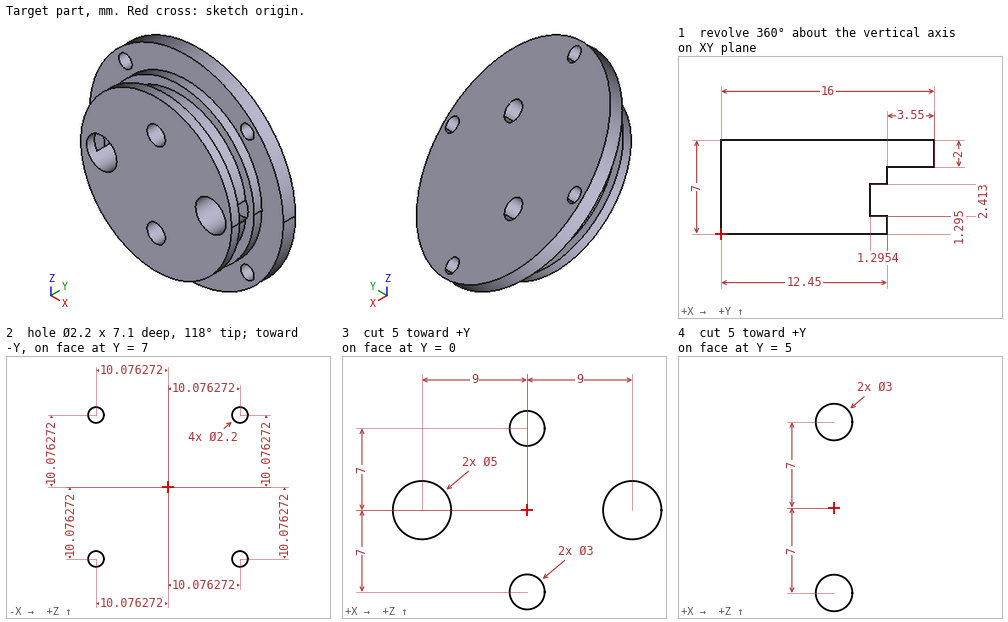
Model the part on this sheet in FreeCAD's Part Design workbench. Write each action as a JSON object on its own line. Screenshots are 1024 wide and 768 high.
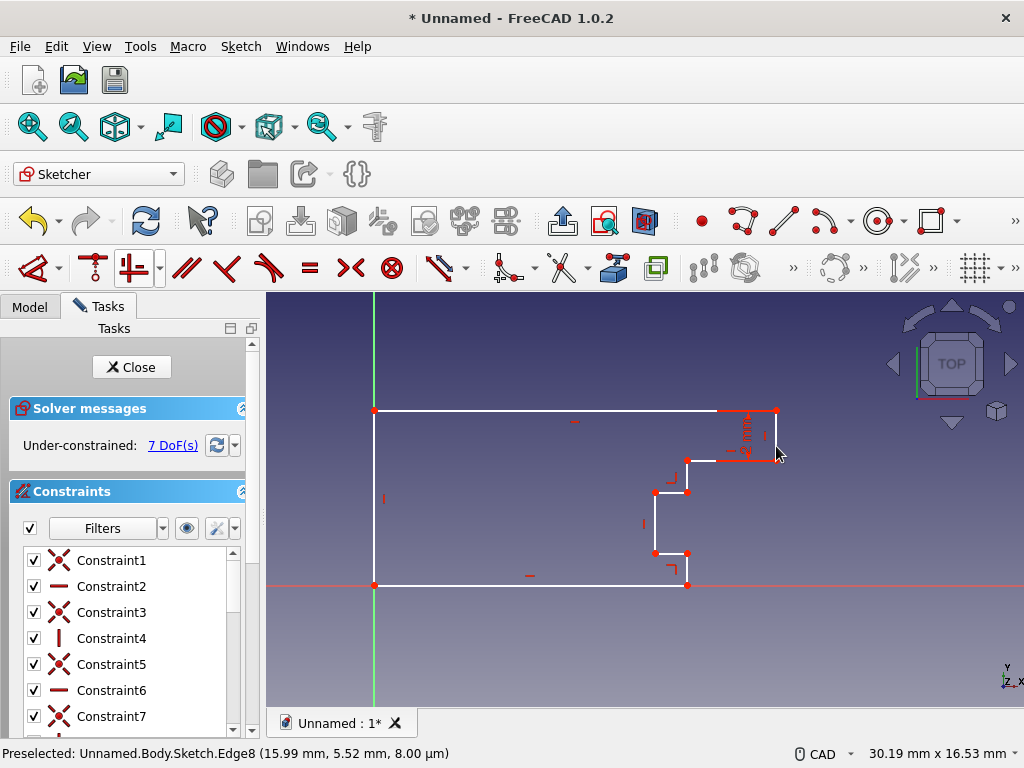
{"action": "left_click", "coordinate": [374, 463]}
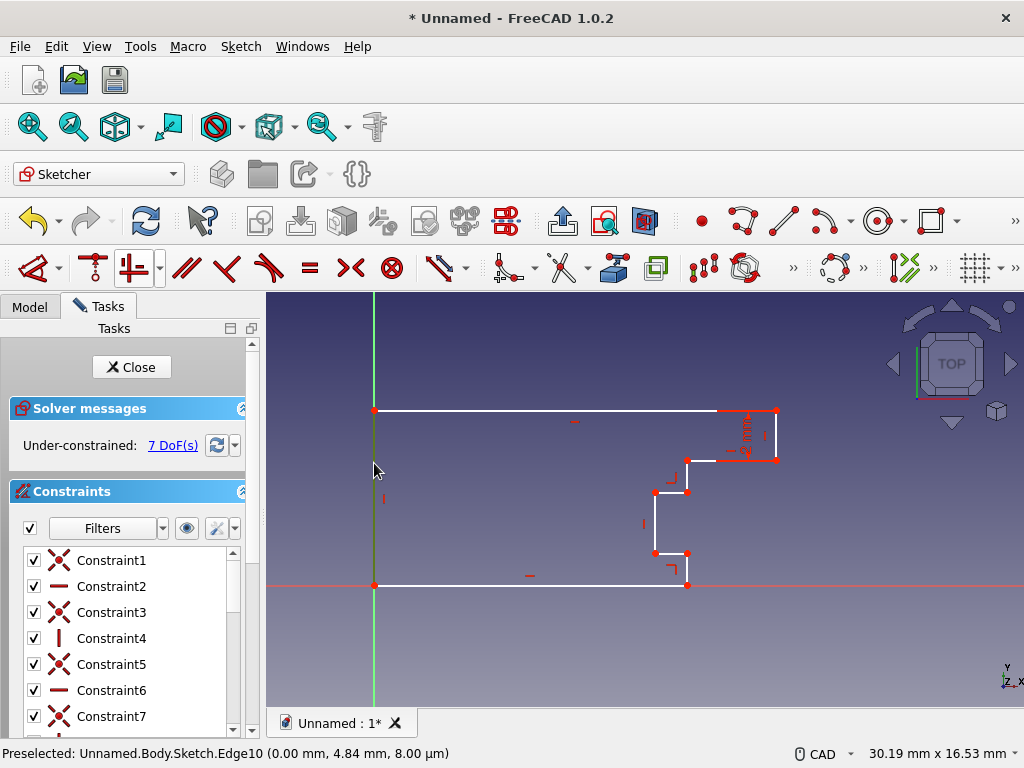
{"action": "left_click", "coordinate": [58, 268]}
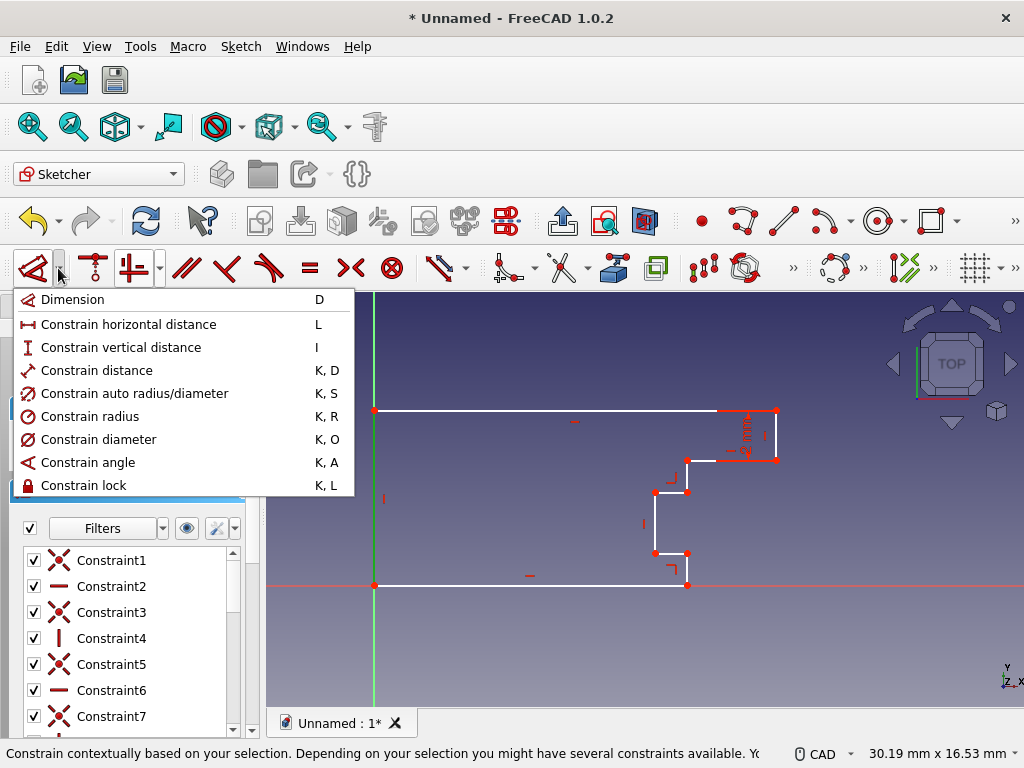
{"action": "left_click", "coordinate": [184, 348]}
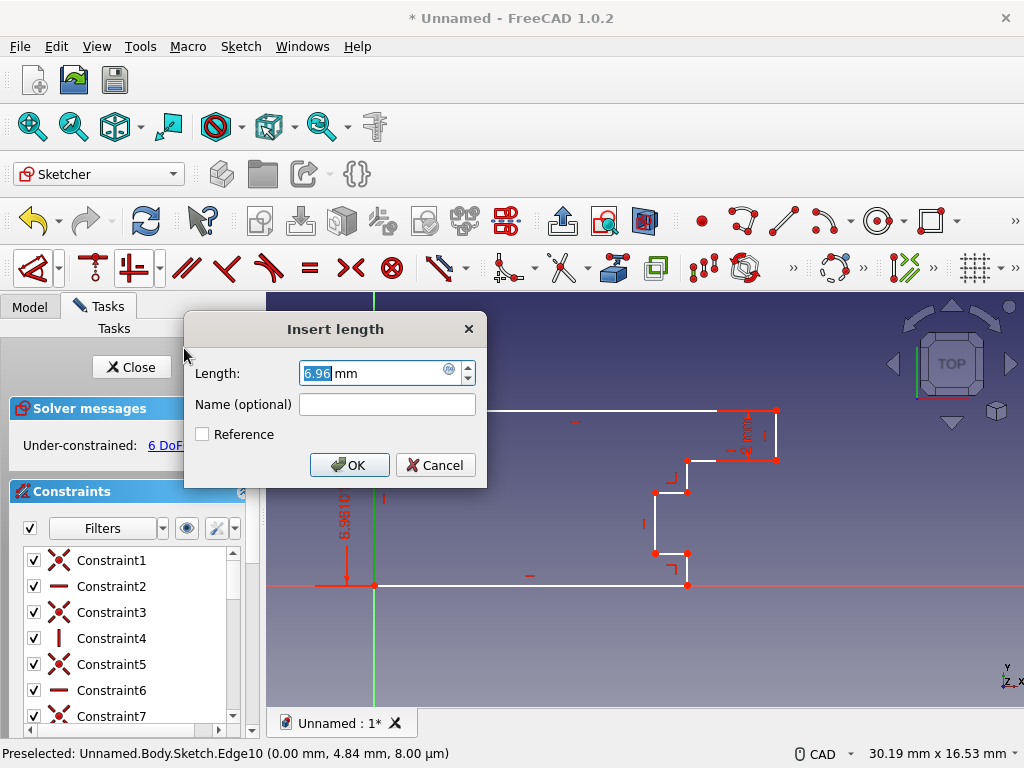
{"action": "type", "text": "7"}
{"action": "key", "text": "Return"}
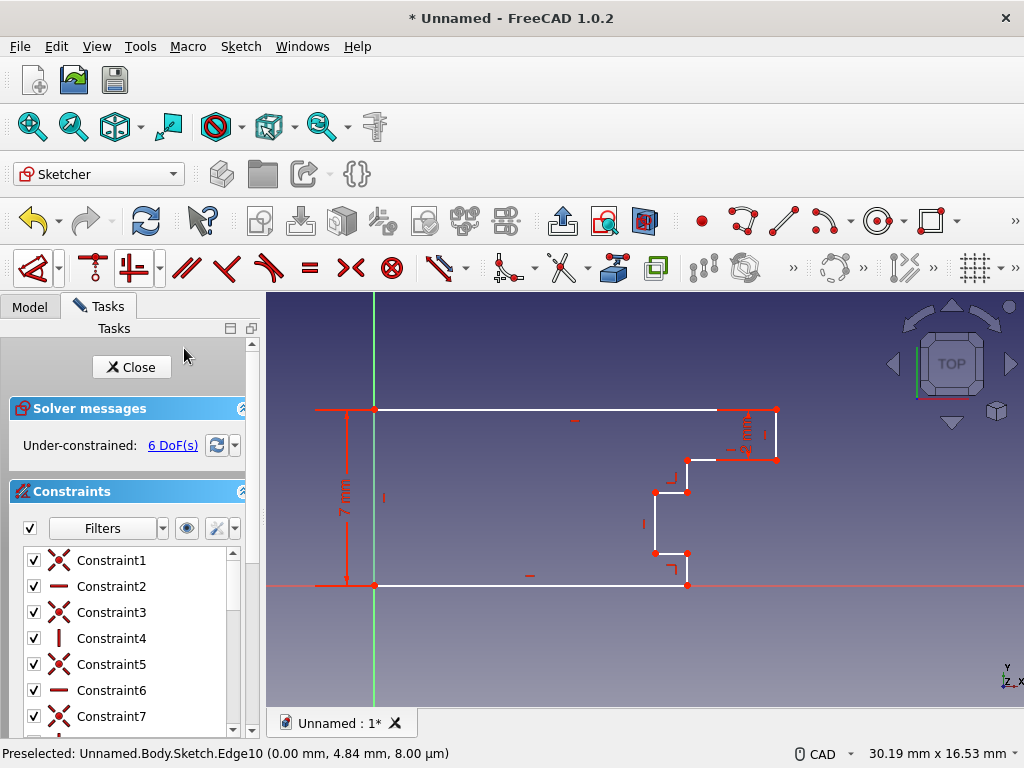
{"action": "left_click", "coordinate": [656, 410]}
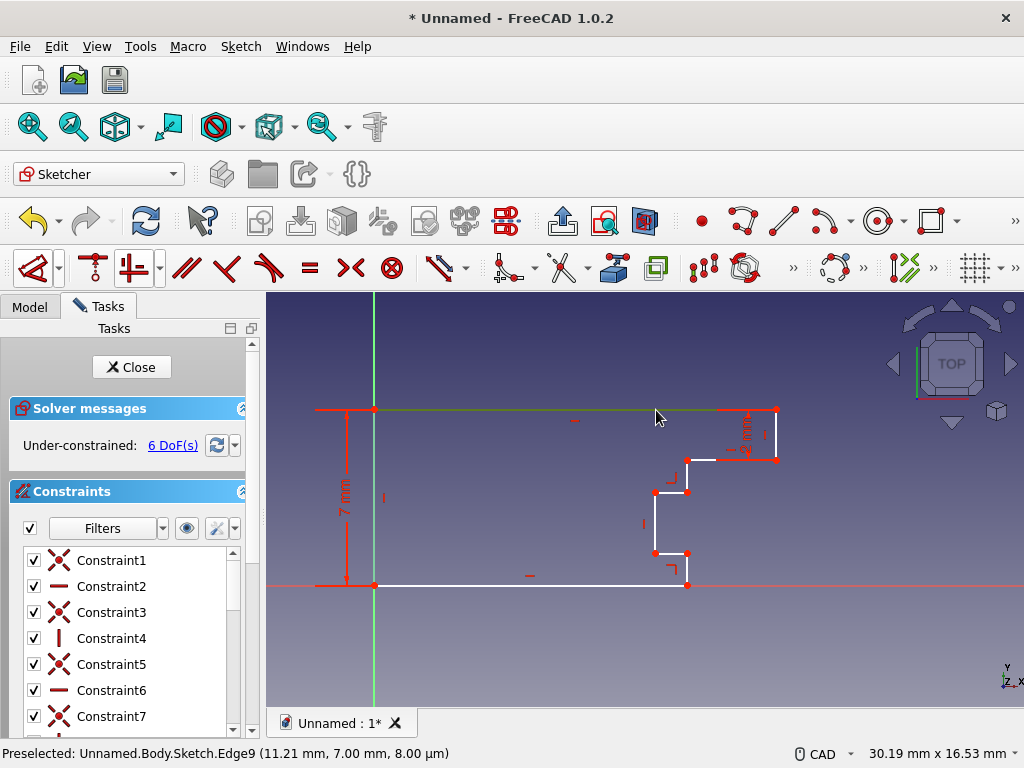
{"action": "left_click", "coordinate": [58, 268]}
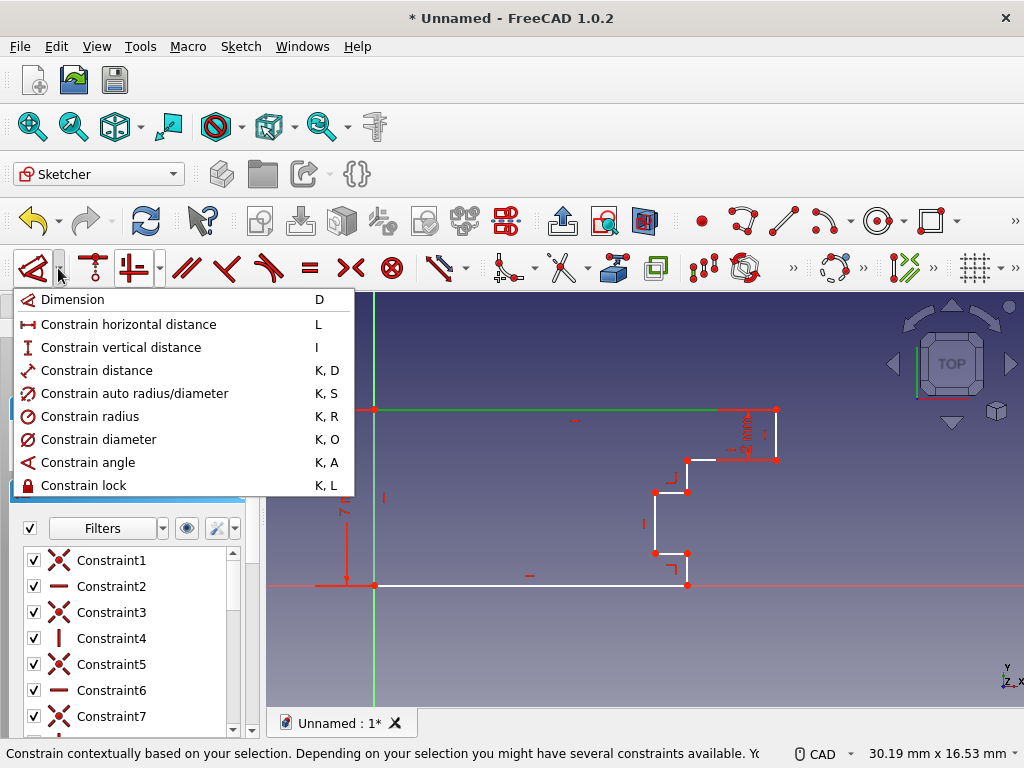
{"action": "left_click", "coordinate": [184, 324]}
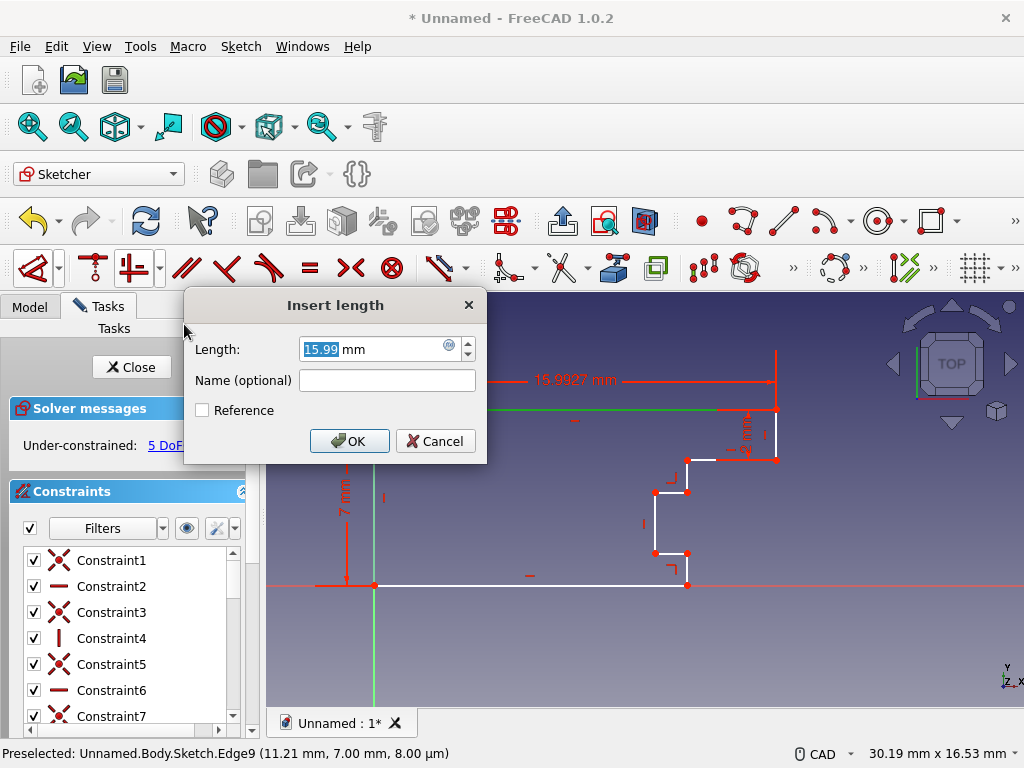
{"action": "type", "text": "16"}
{"action": "key", "text": "Return"}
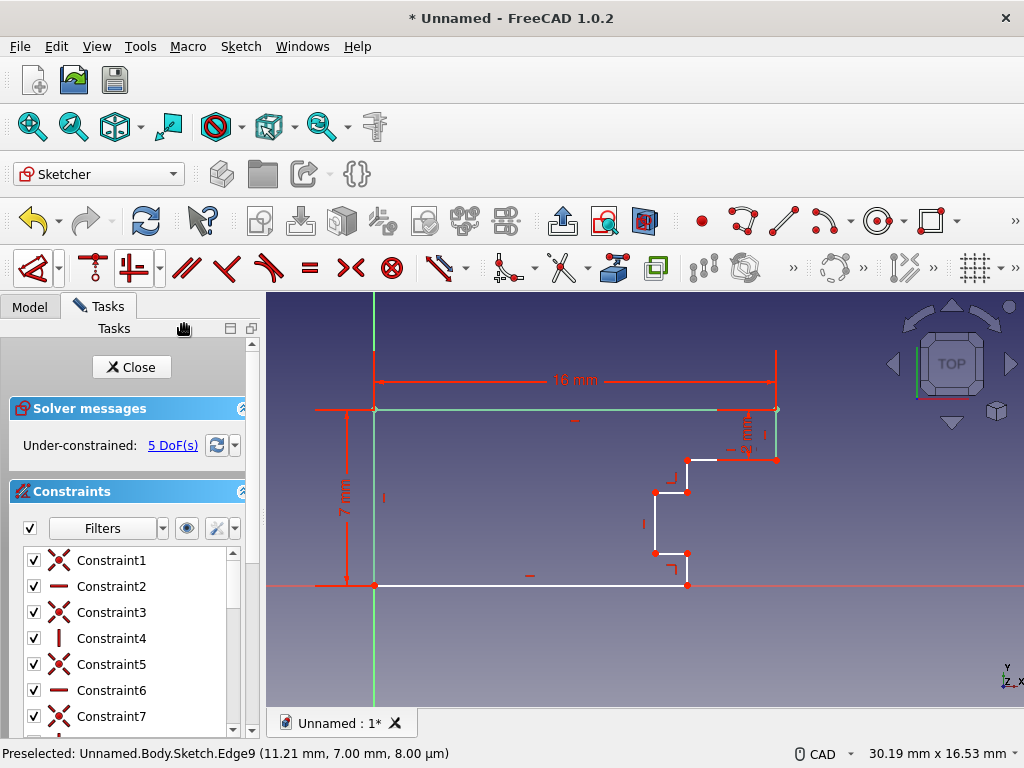
{"action": "left_click", "coordinate": [714, 460]}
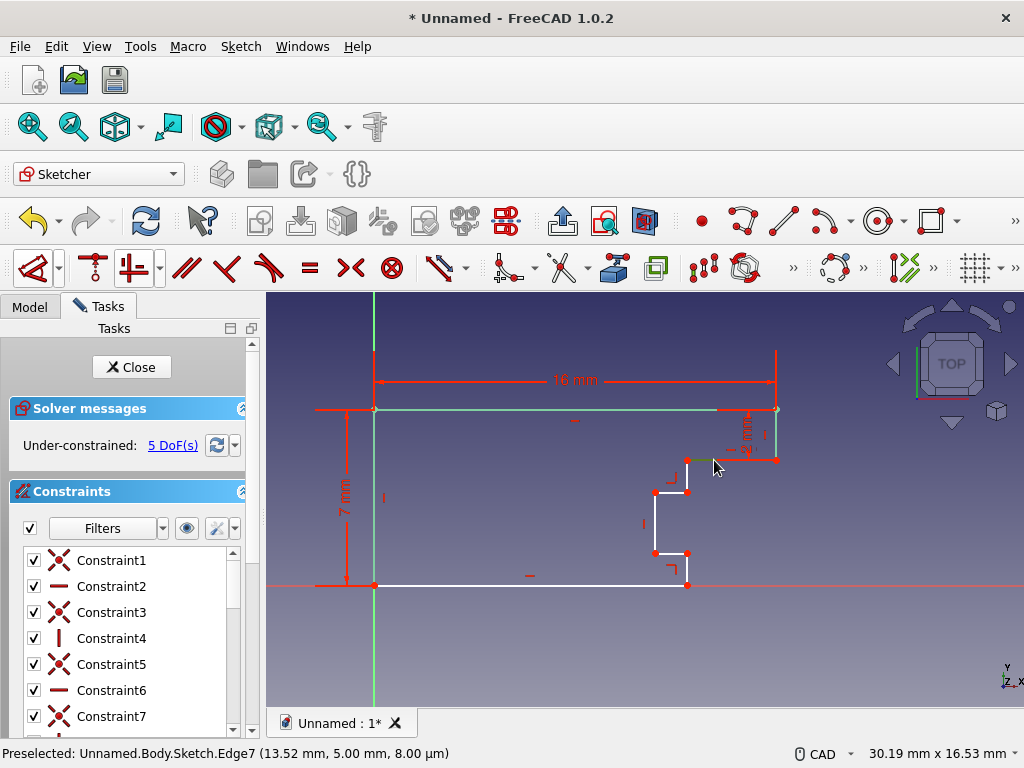
{"action": "left_click", "coordinate": [58, 268]}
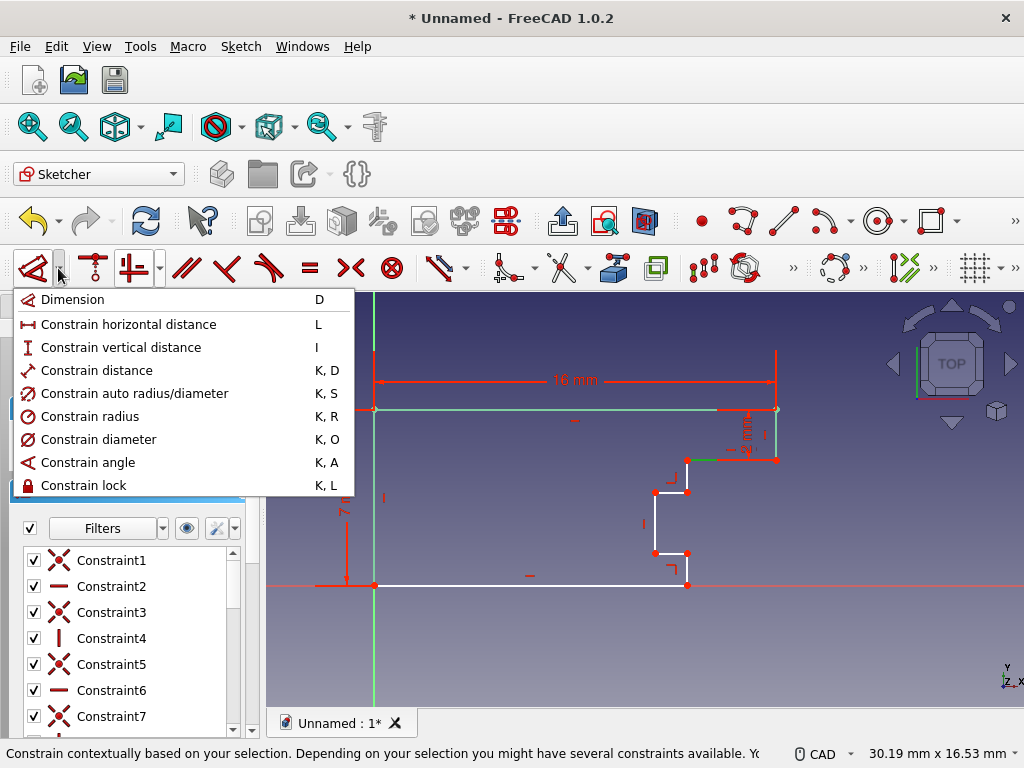
{"action": "left_click", "coordinate": [184, 324]}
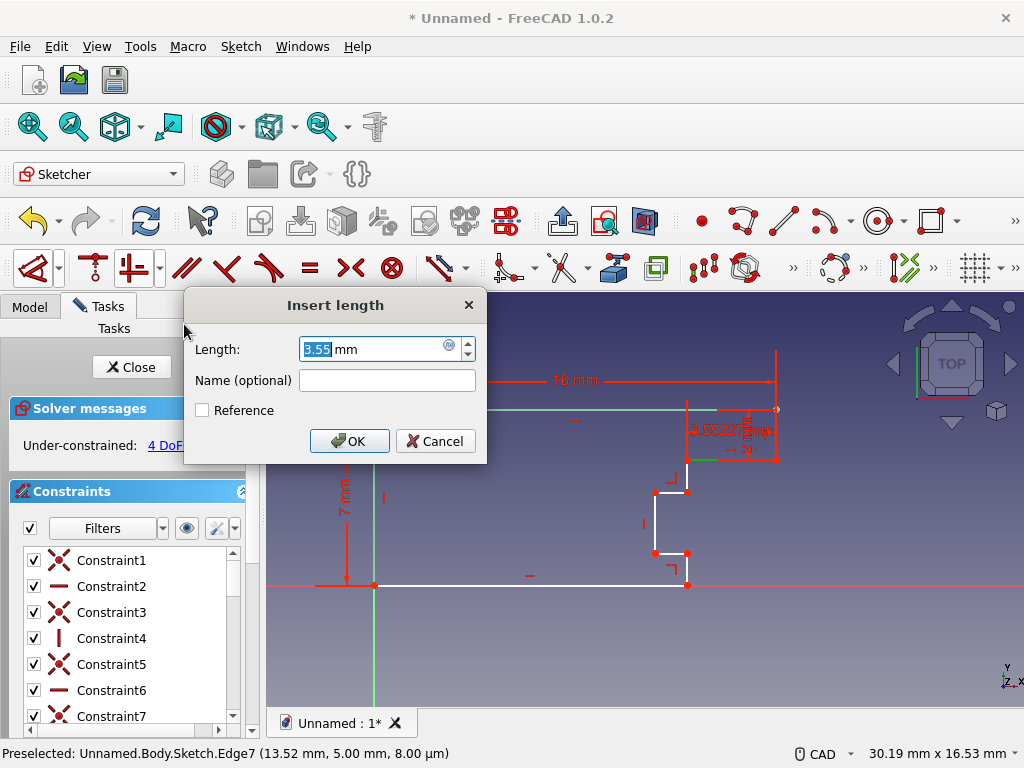
{"action": "type", "text": "3.55"}
{"action": "key", "text": "Return"}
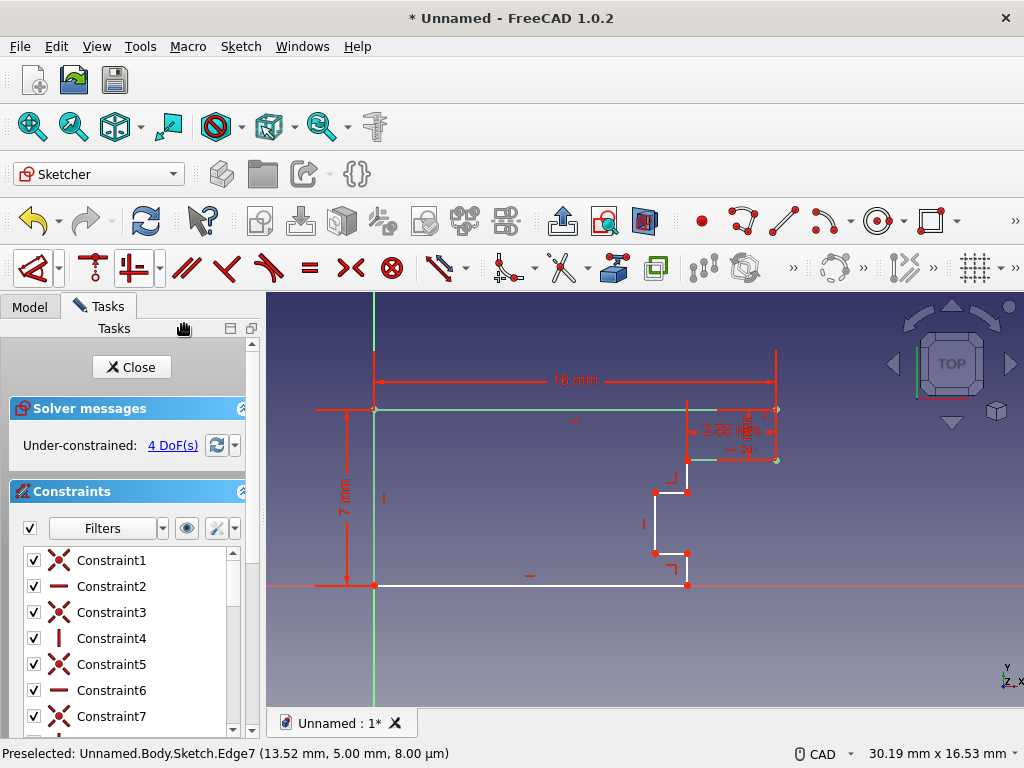
{"action": "left_click", "coordinate": [468, 586]}